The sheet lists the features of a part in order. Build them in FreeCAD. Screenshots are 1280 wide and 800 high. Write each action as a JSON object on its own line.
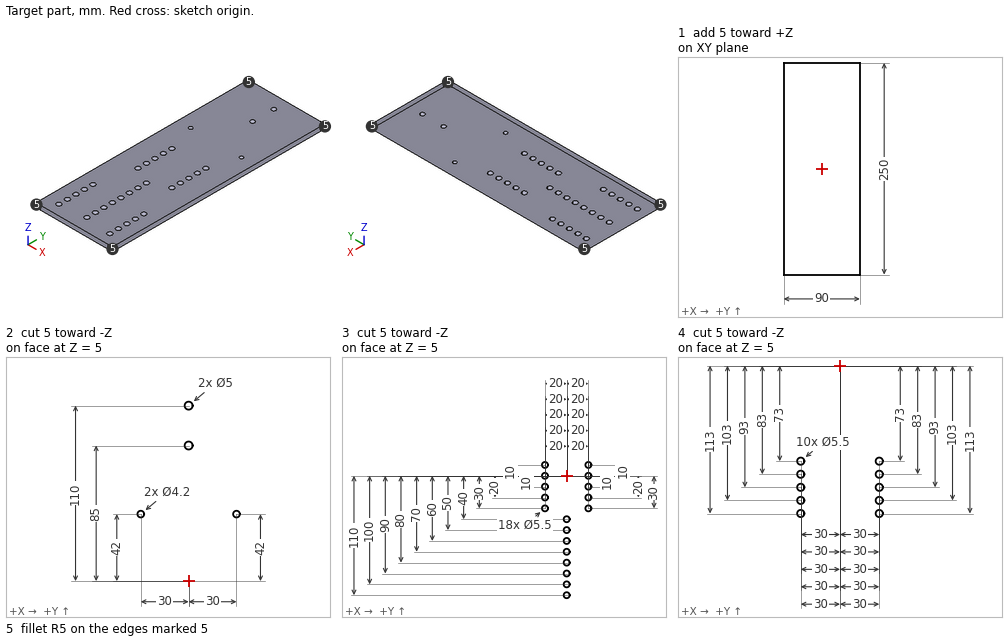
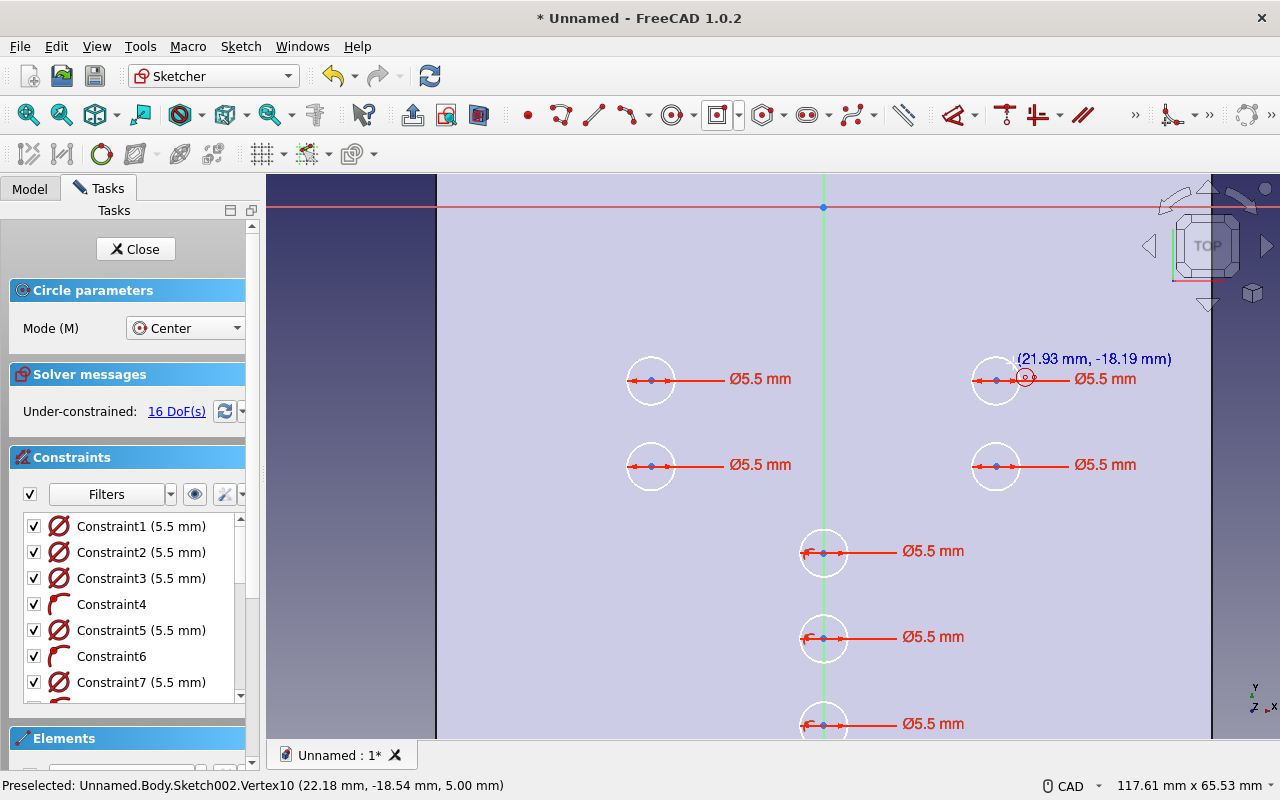
{"action": "left_click", "coordinate": [651, 293]}
{"action": "mouse_move", "coordinate": [668, 277]}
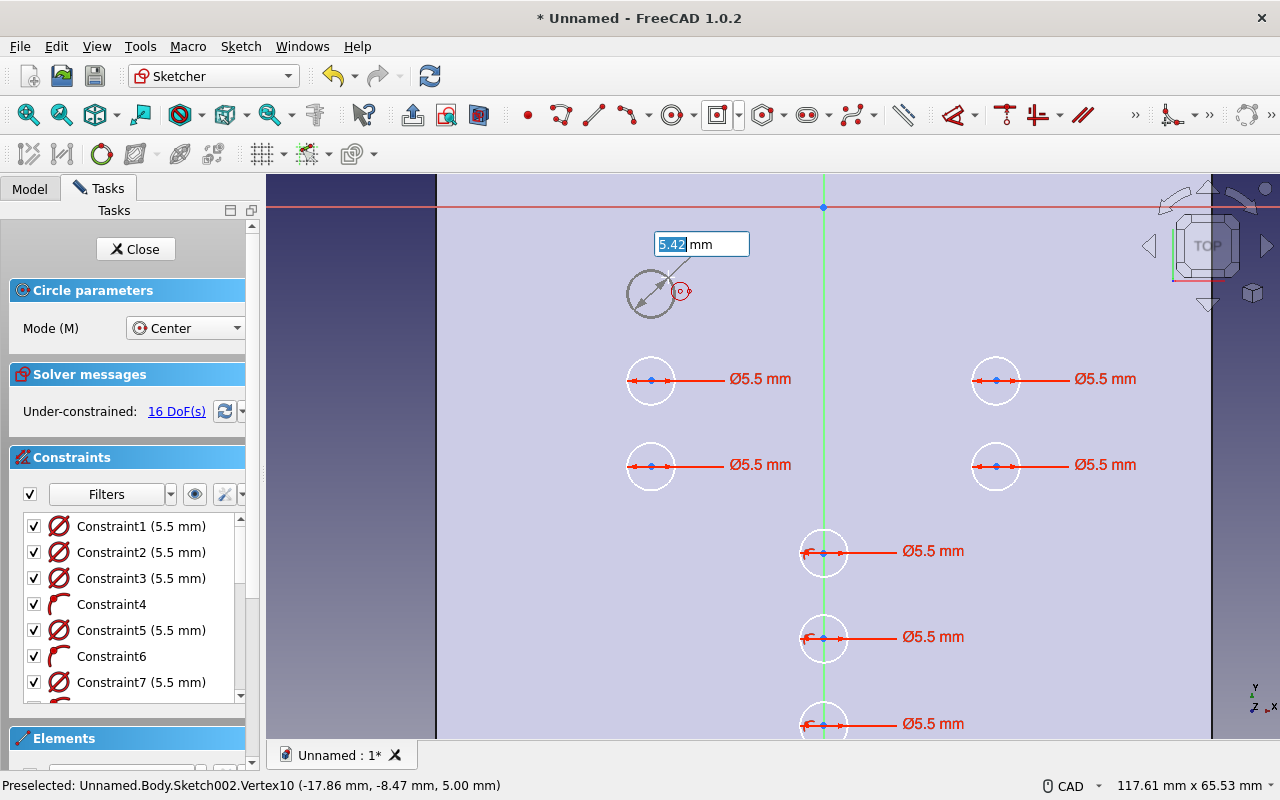
{"action": "type", "text": "5.5"}
{"action": "key", "text": "Return"}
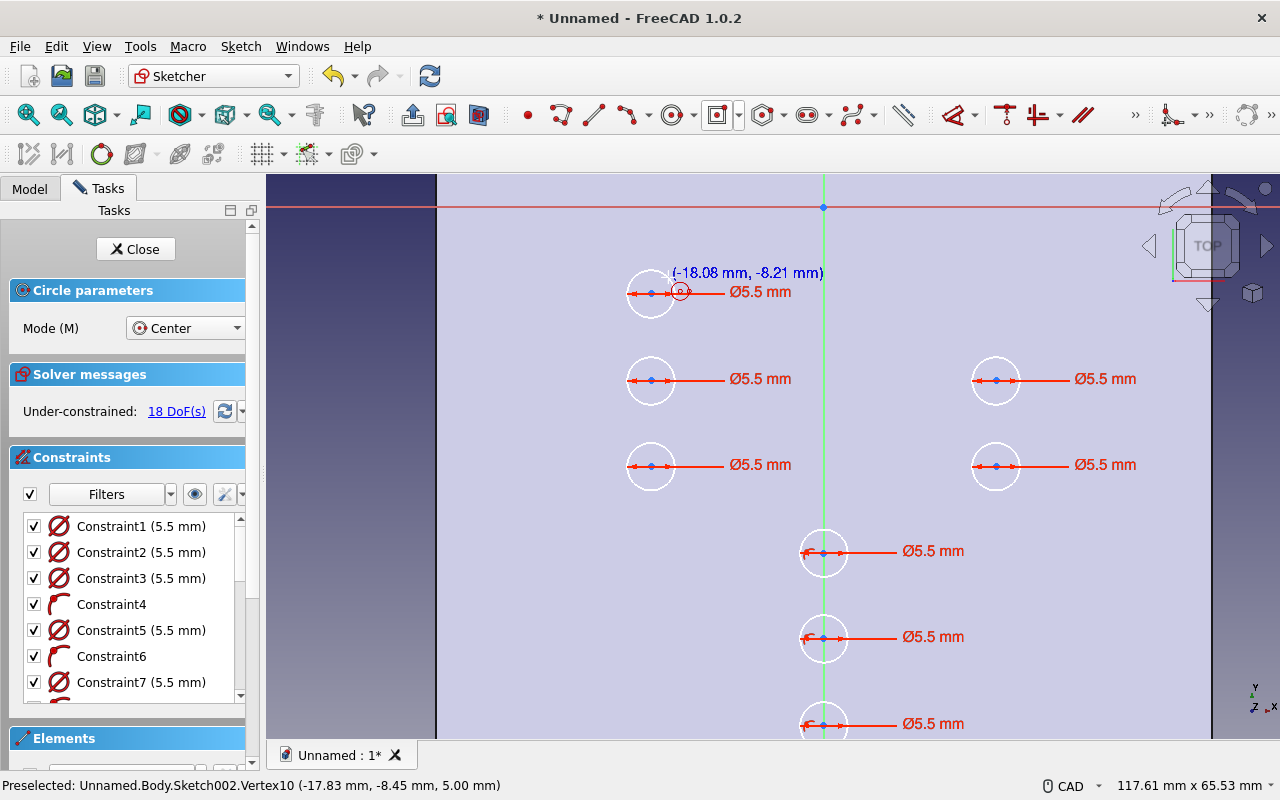
{"action": "left_click", "coordinate": [996, 293]}
{"action": "mouse_move", "coordinate": [1013, 277]}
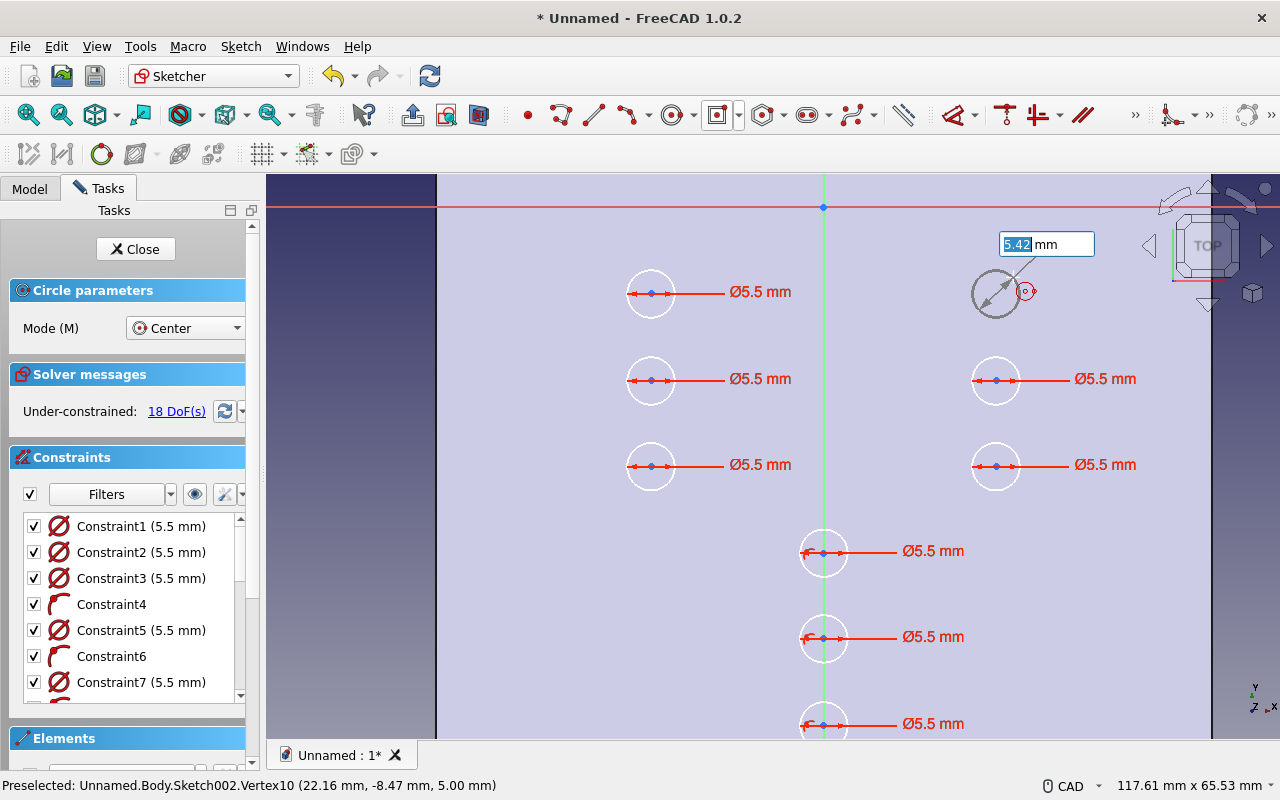
{"action": "type", "text": "5.5"}
{"action": "key", "text": "Return"}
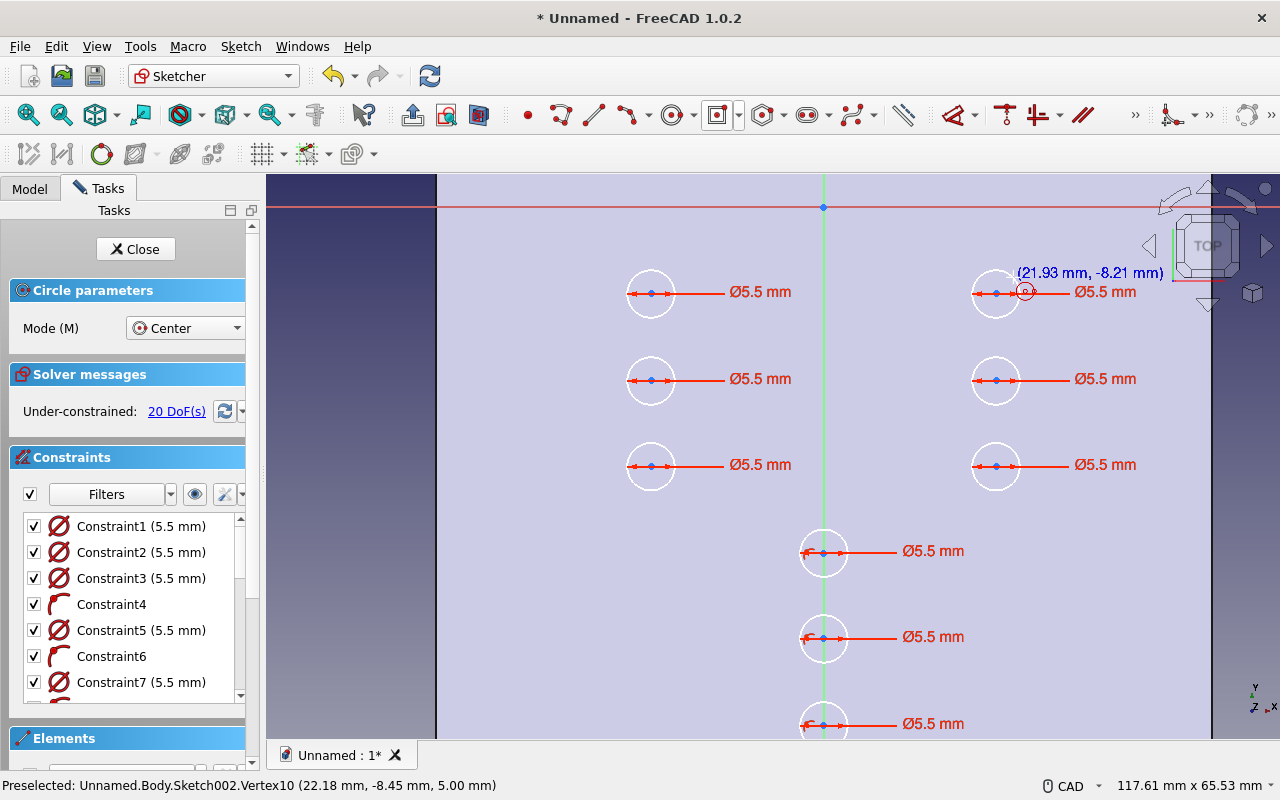
{"action": "left_click", "coordinate": [651, 207]}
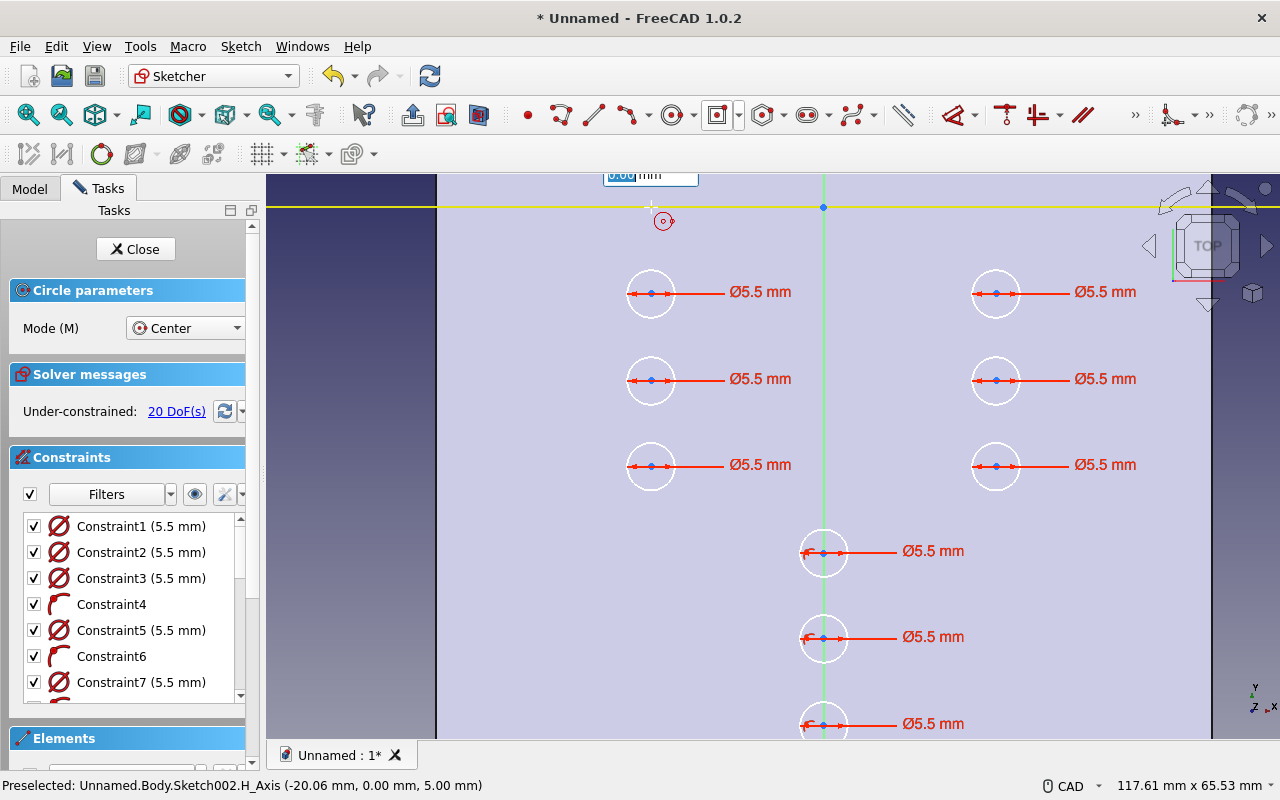
{"action": "scroll", "coordinate": [653, 378], "scroll_direction": "down", "scroll_amount": 6}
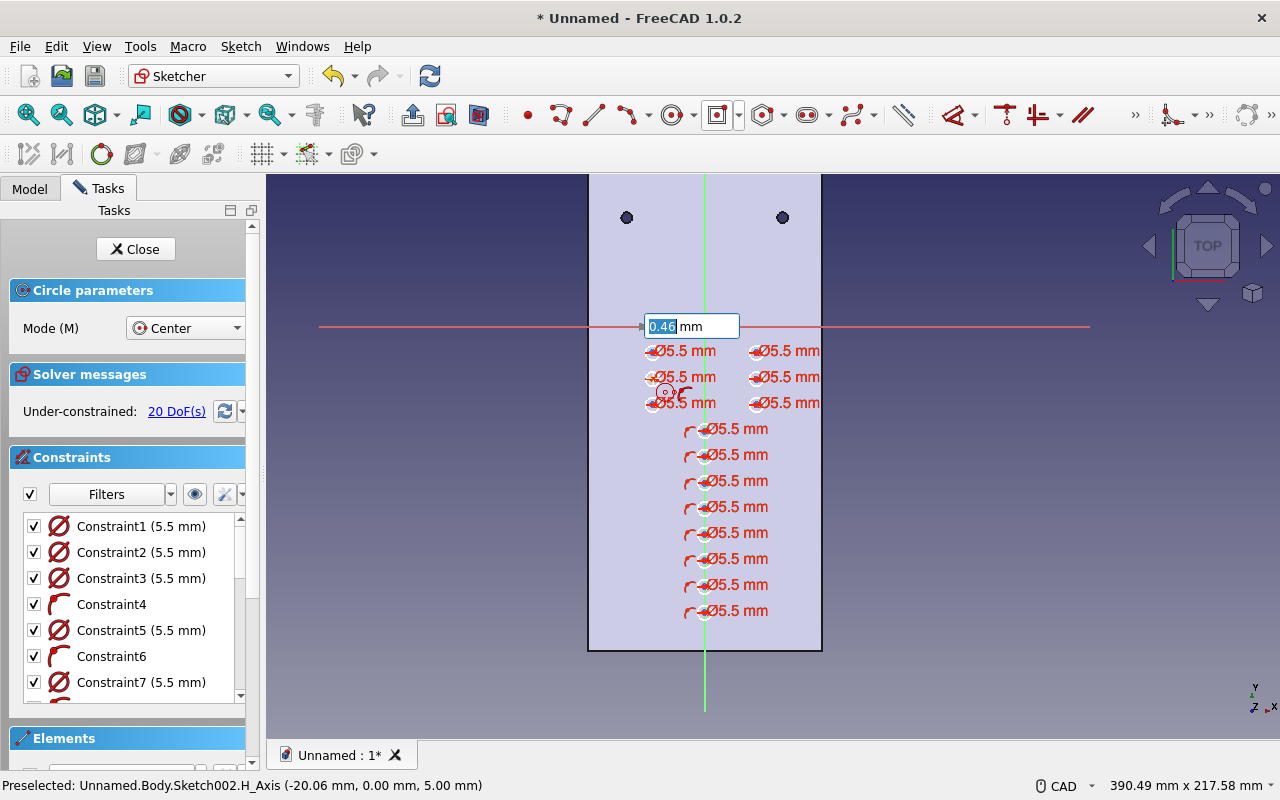
{"action": "scroll", "coordinate": [658, 322], "scroll_direction": "up", "scroll_amount": 6}
{"action": "mouse_move", "coordinate": [657, 321]}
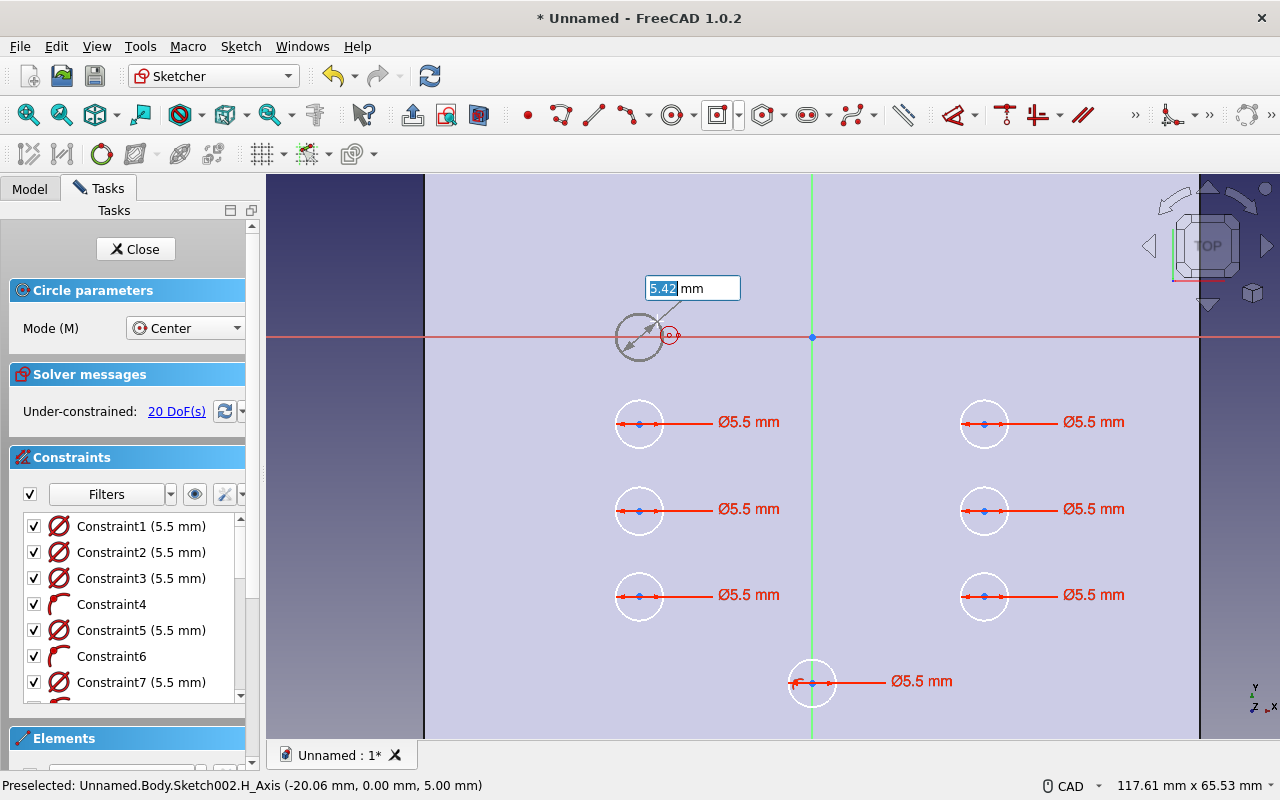
{"action": "type", "text": "5.5"}
{"action": "key", "text": "Return"}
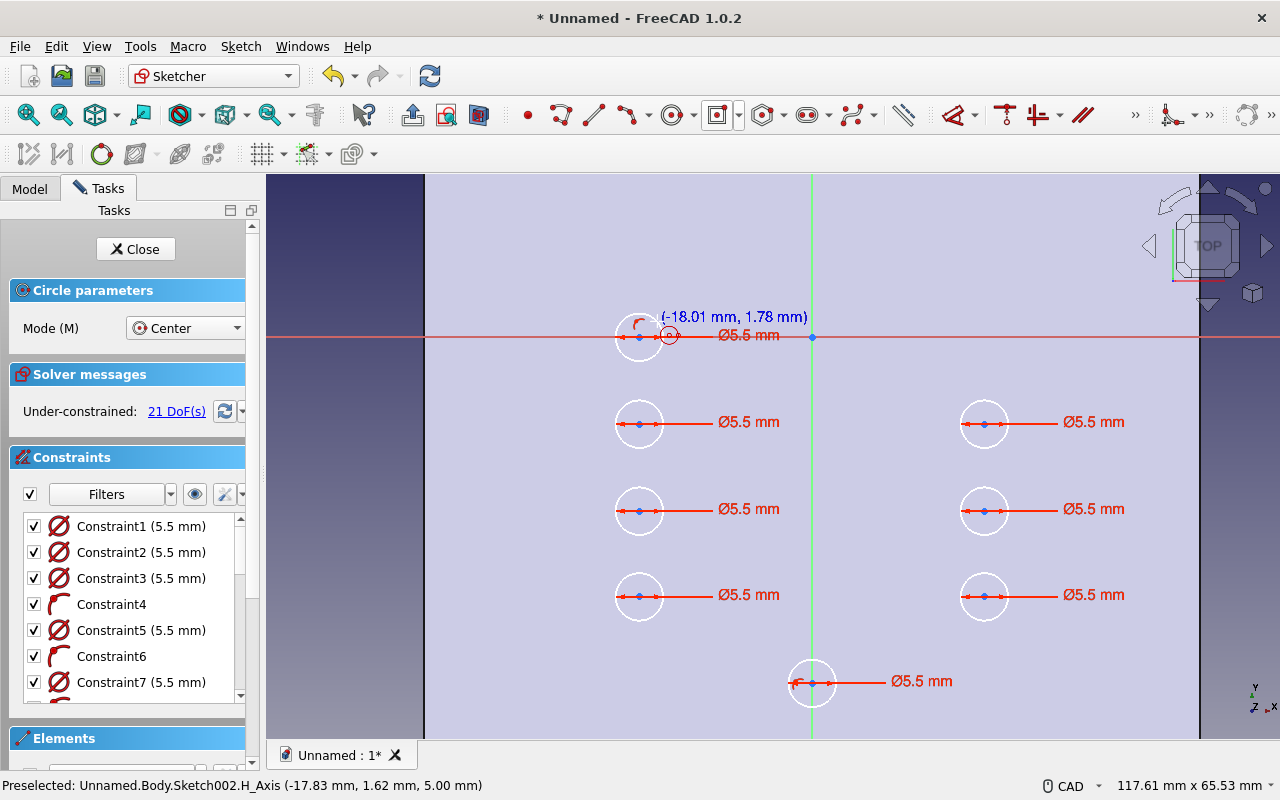
{"action": "left_click", "coordinate": [985, 337]}
{"action": "mouse_move", "coordinate": [1001, 321]}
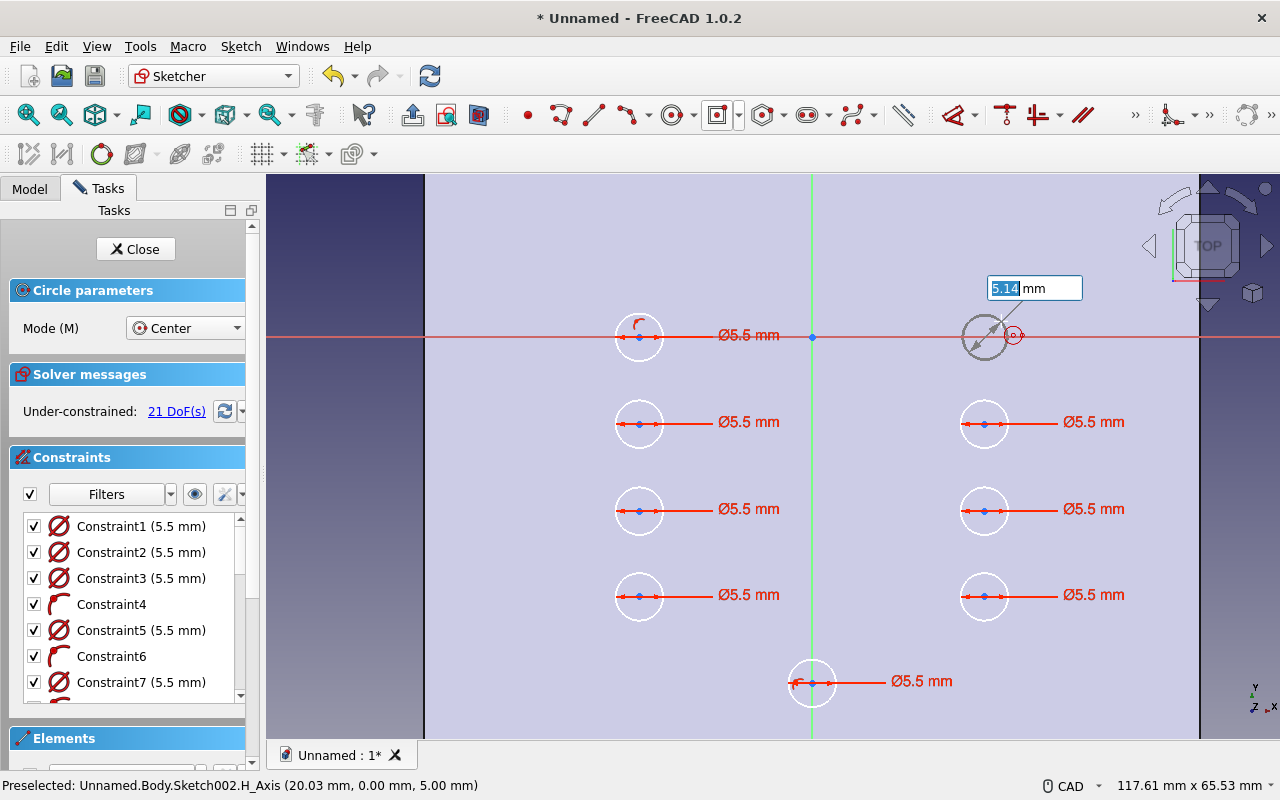
{"action": "type", "text": "5.5"}
{"action": "key", "text": "Return"}